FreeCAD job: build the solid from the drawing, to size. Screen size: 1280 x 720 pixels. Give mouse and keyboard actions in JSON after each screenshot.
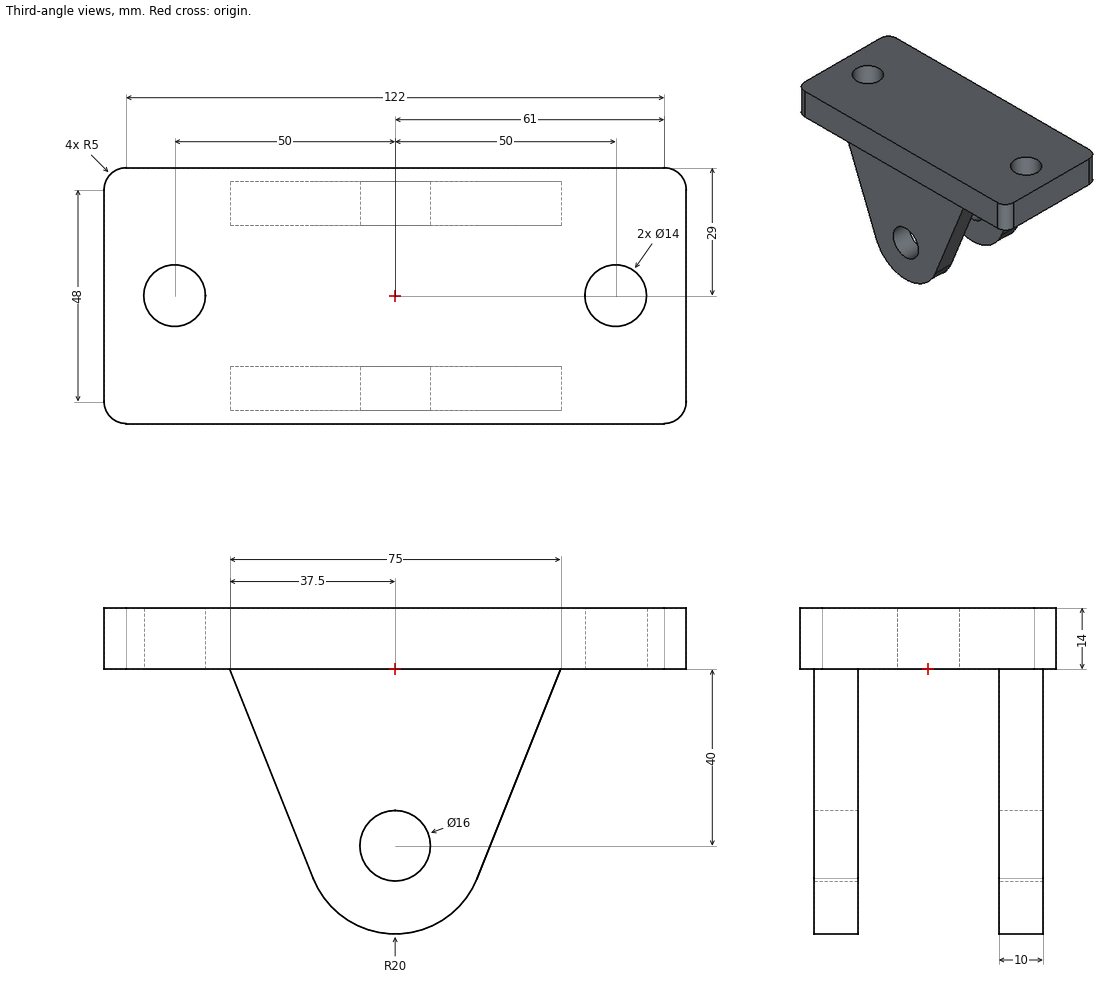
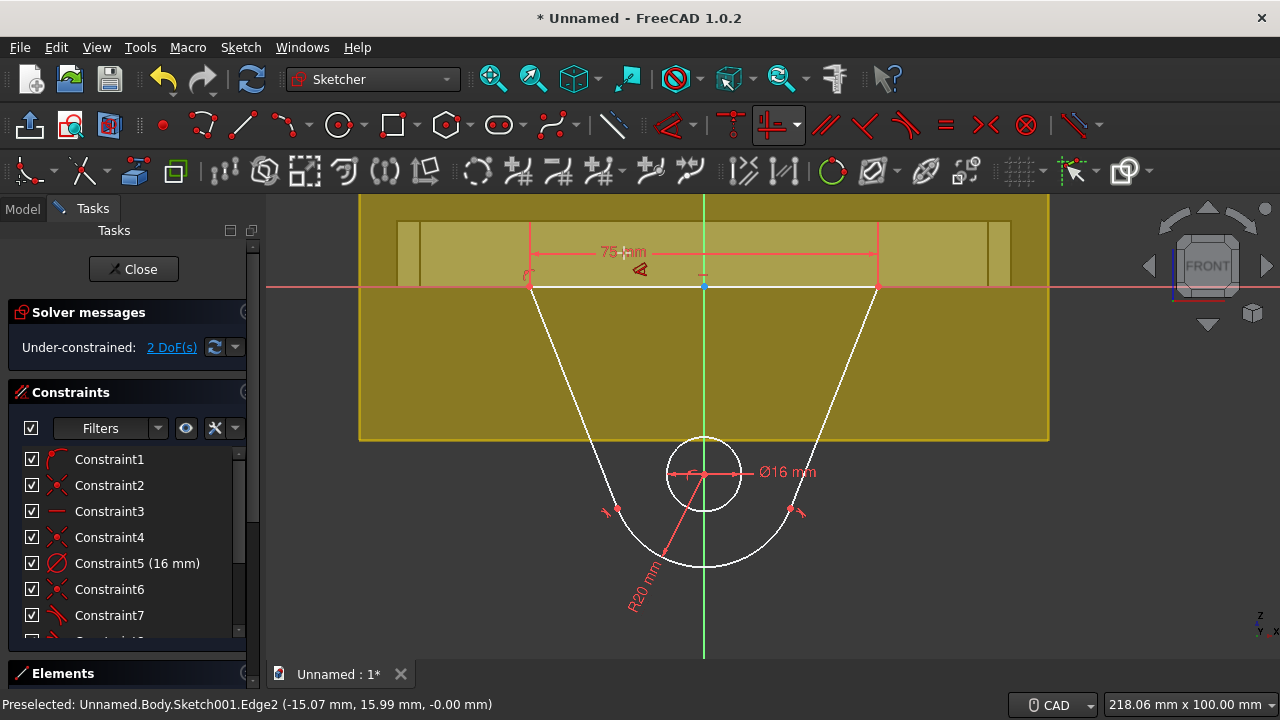
{"action": "left_click", "coordinate": [704, 474]}
{"action": "left_click", "coordinate": [738, 380]}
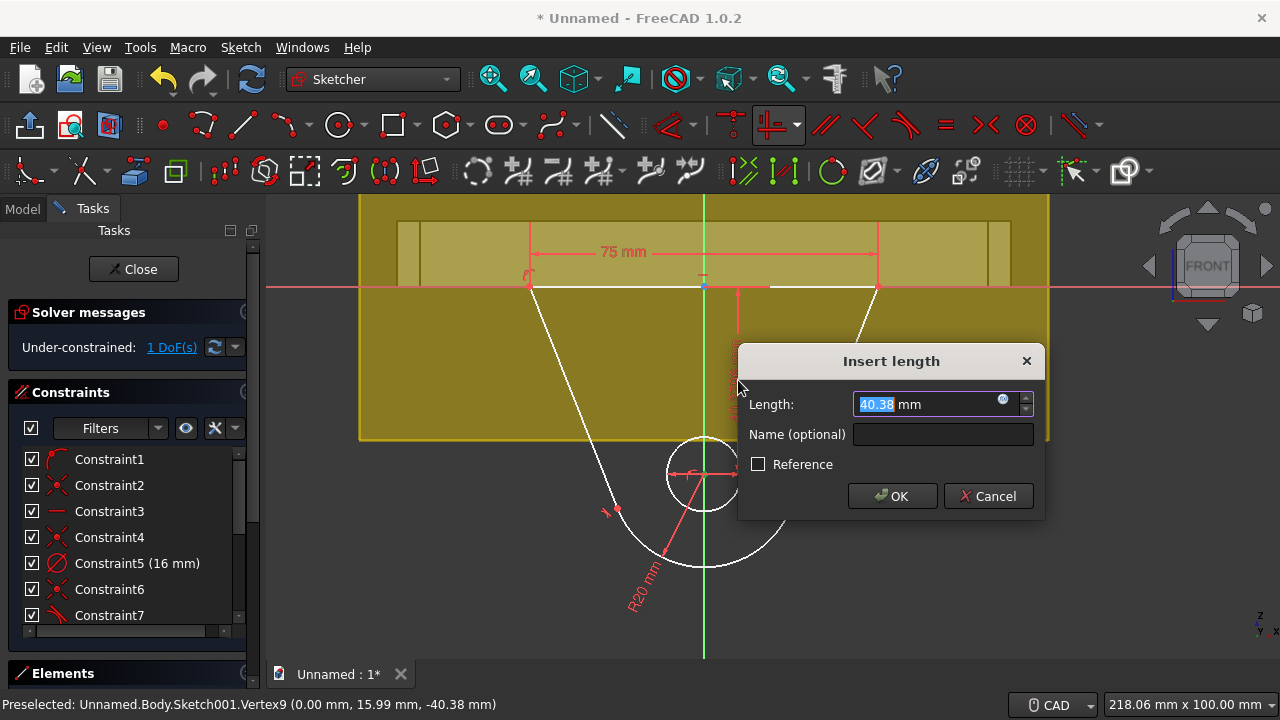
{"action": "type", "text": "40"}
{"action": "key", "text": "Return"}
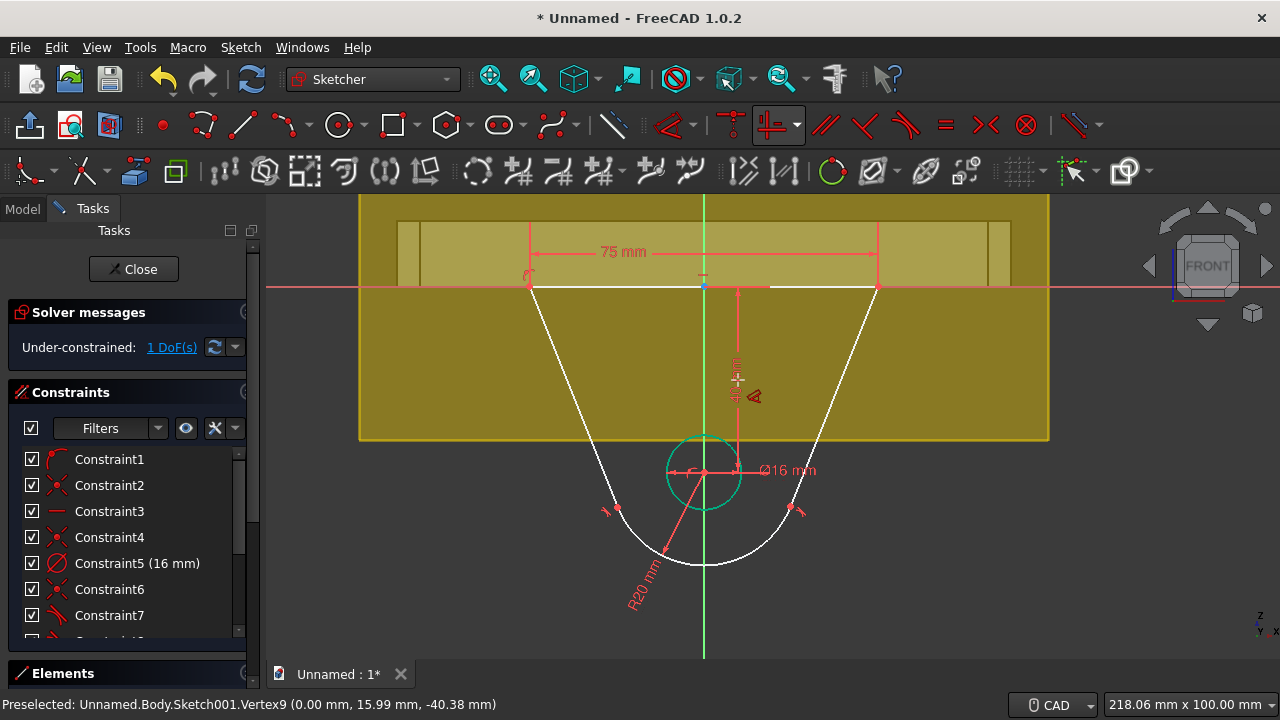
{"action": "left_click", "coordinate": [530, 287]}
{"action": "left_click", "coordinate": [617, 321]}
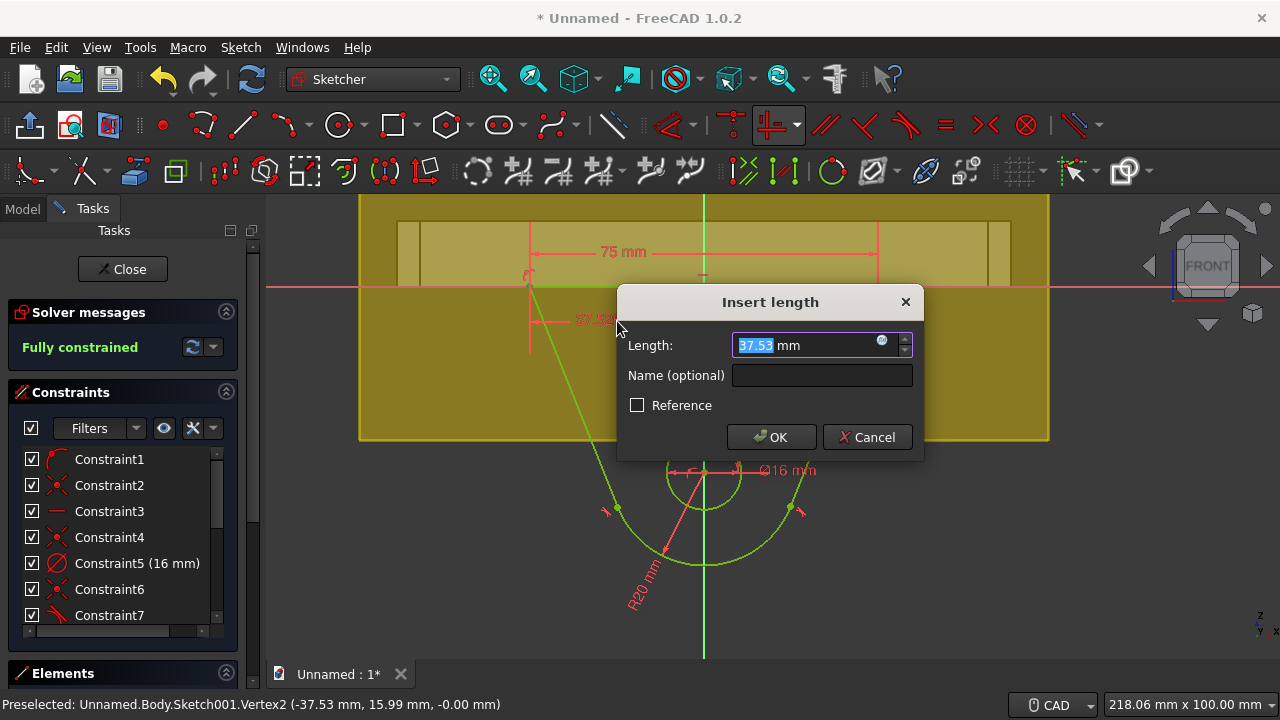
{"action": "type", "text": "37.5"}
{"action": "key", "text": "Return"}
{"action": "key", "text": "Escape"}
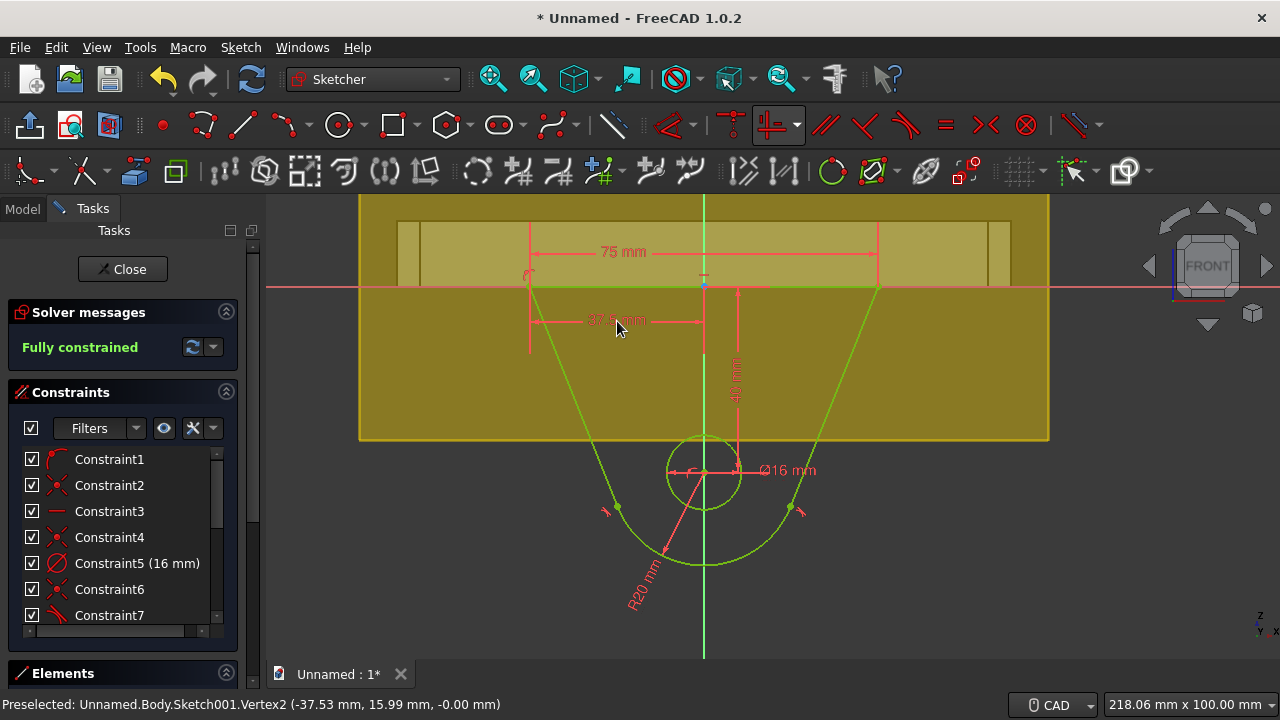
{"action": "left_click", "coordinate": [123, 269]}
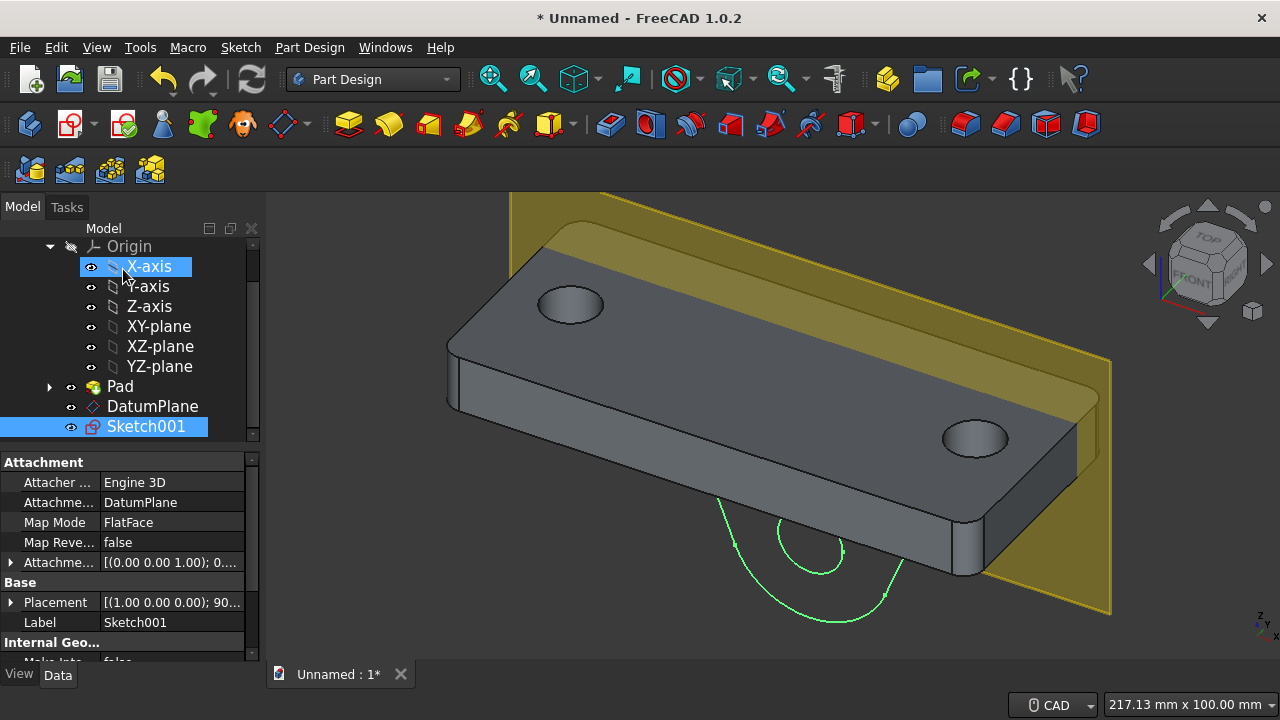
{"action": "left_click", "coordinate": [350, 124]}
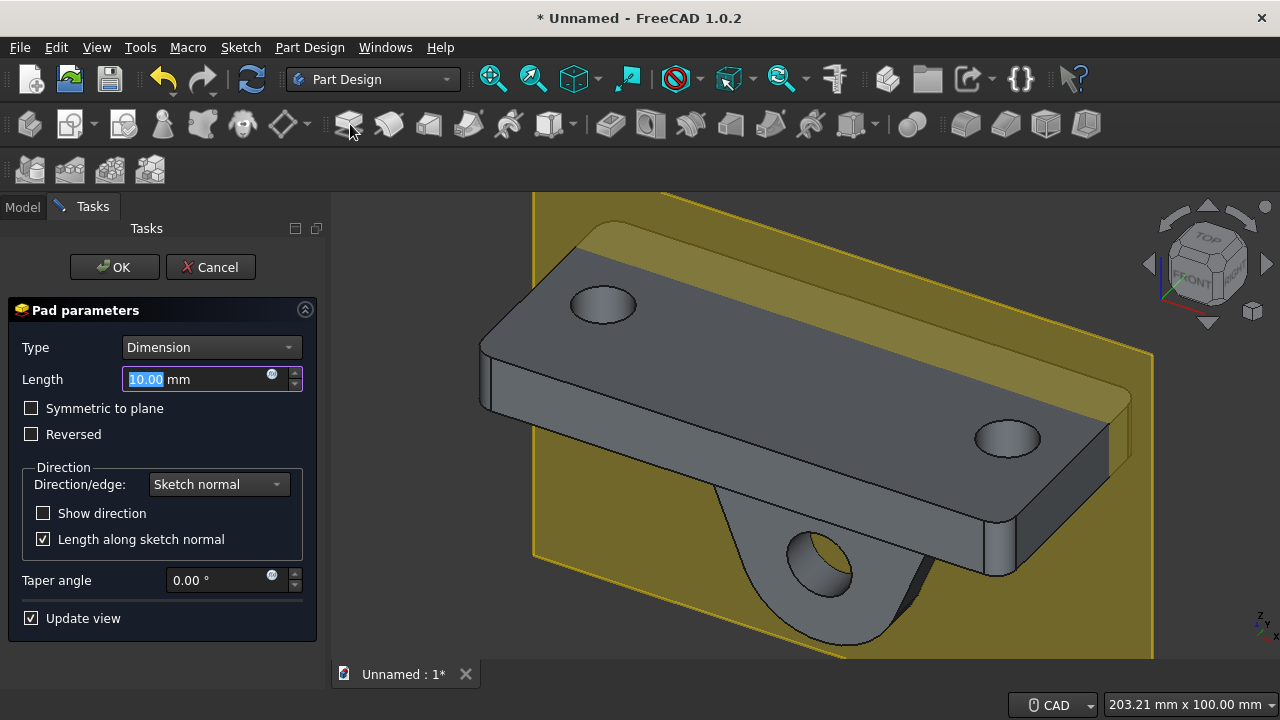
{"action": "type", "text": "10"}
{"action": "key", "text": "Tab"}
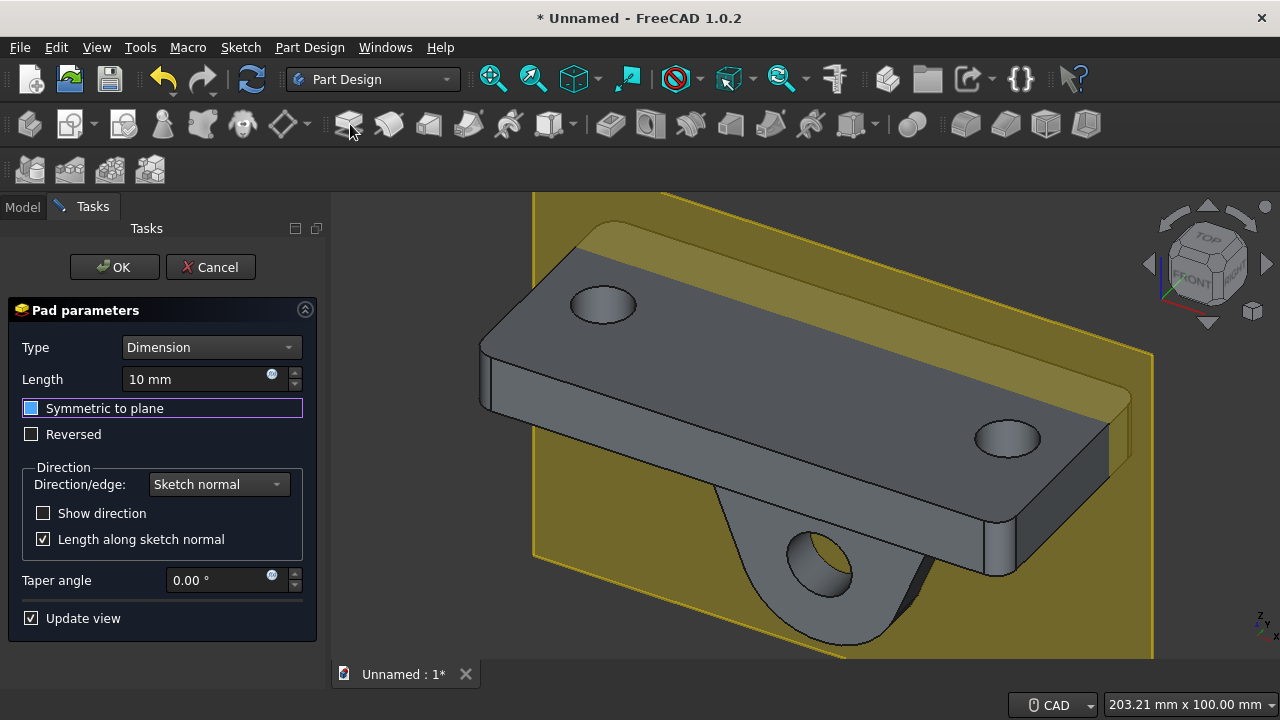
{"action": "left_click", "coordinate": [30, 434]}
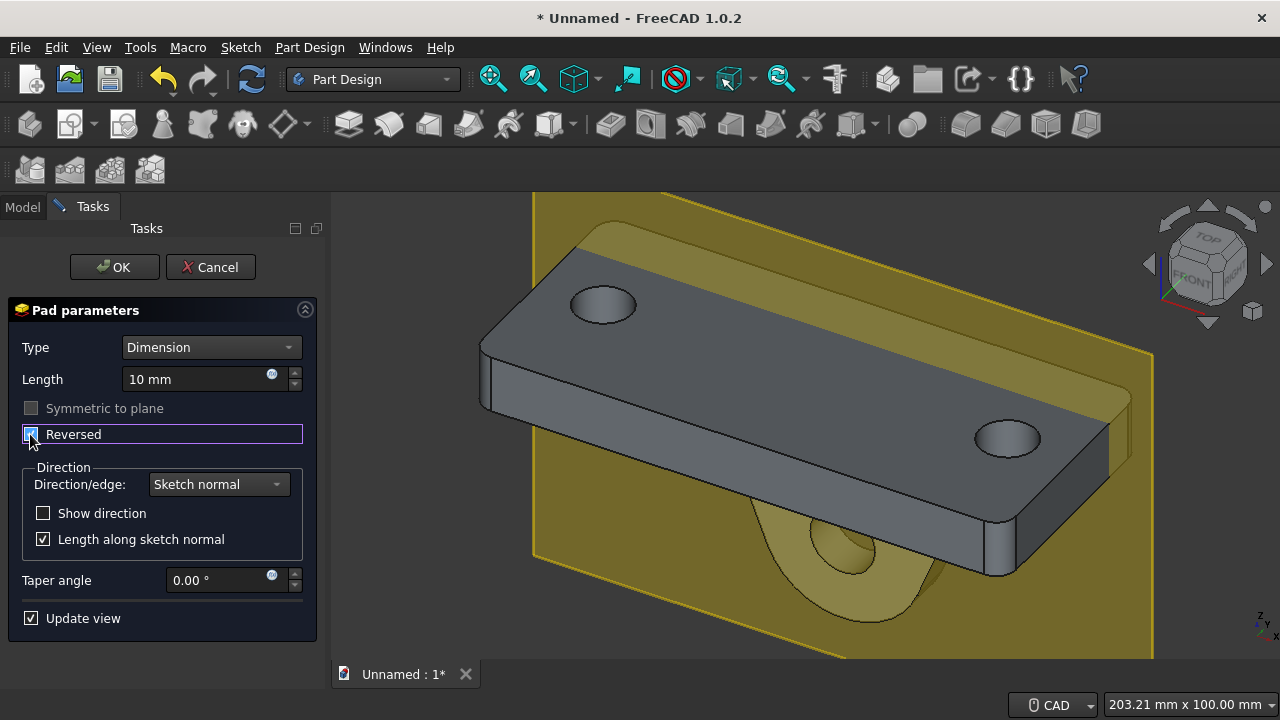
{"action": "left_click", "coordinate": [115, 267]}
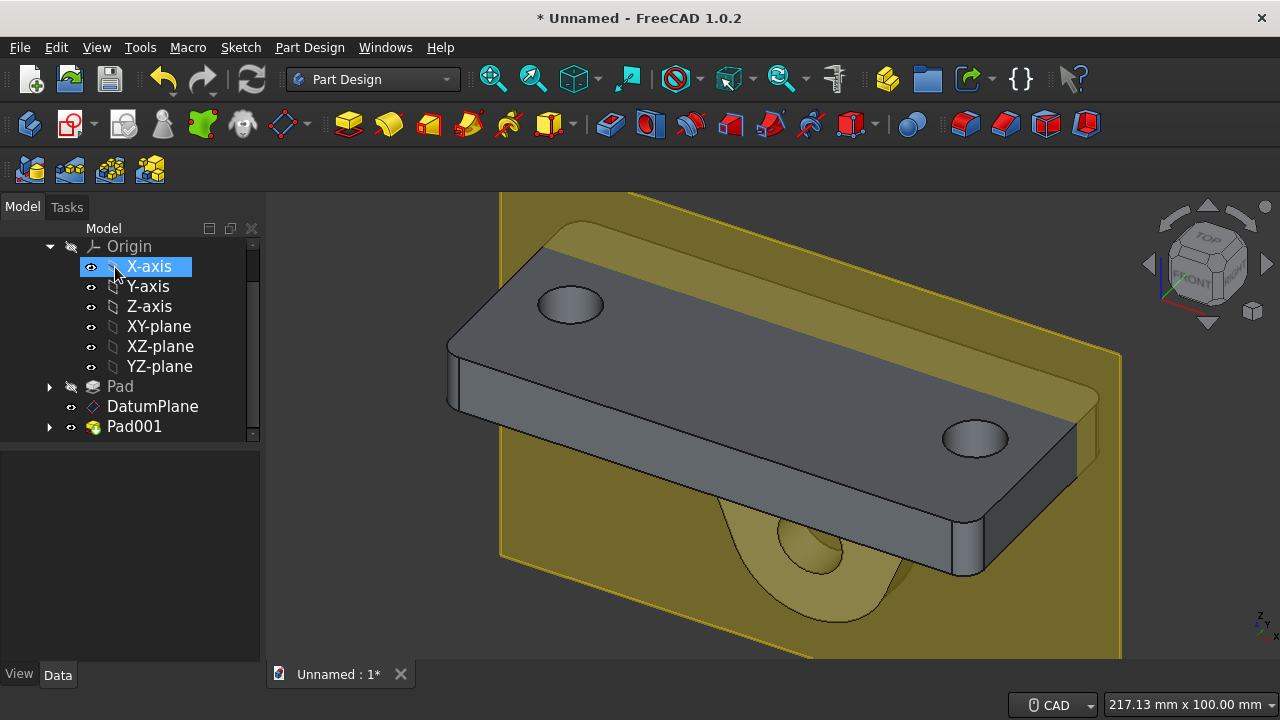
{"action": "left_click", "coordinate": [116, 407]}
{"action": "key", "text": "space"}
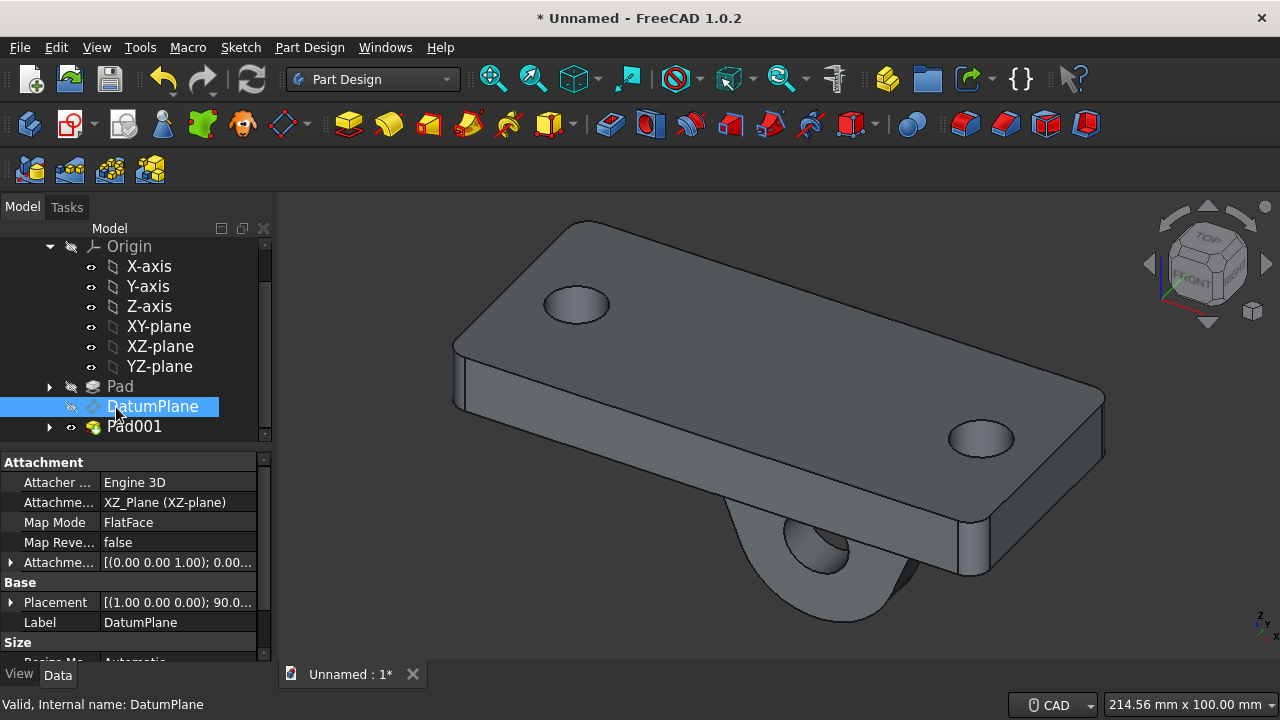
{"action": "left_click", "coordinate": [494, 80]}